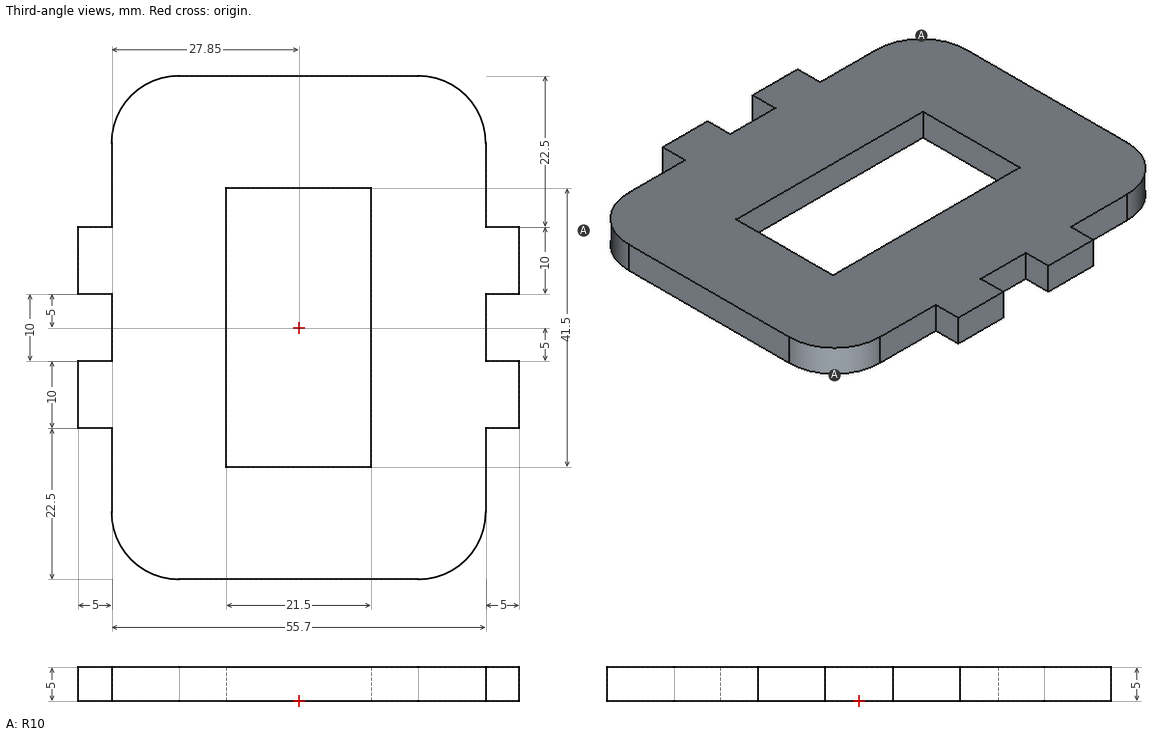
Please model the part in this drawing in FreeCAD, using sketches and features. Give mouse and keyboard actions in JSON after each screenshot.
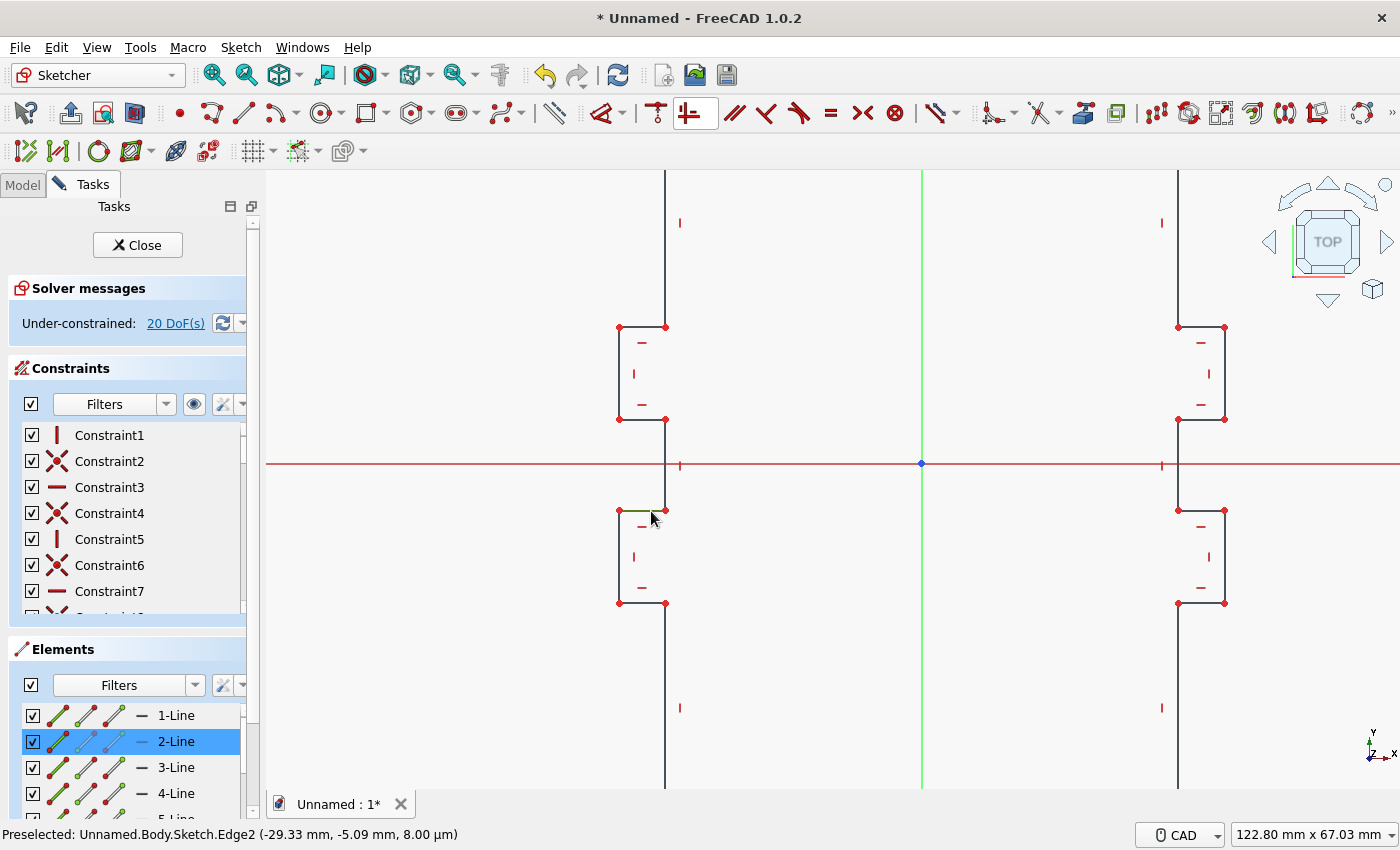
{"action": "key", "text": "l"}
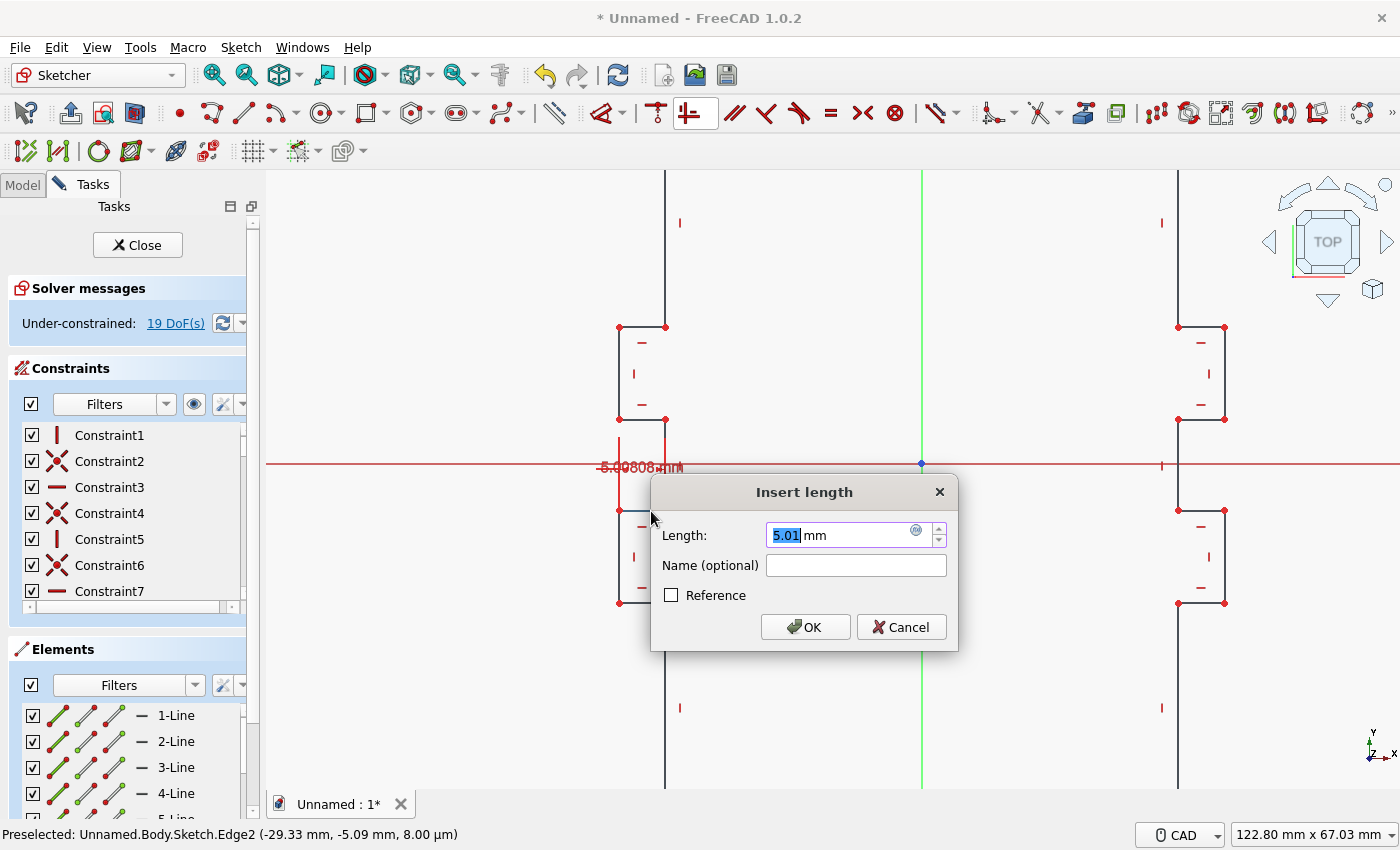
{"action": "type", "text": "5"}
{"action": "key", "text": "Return"}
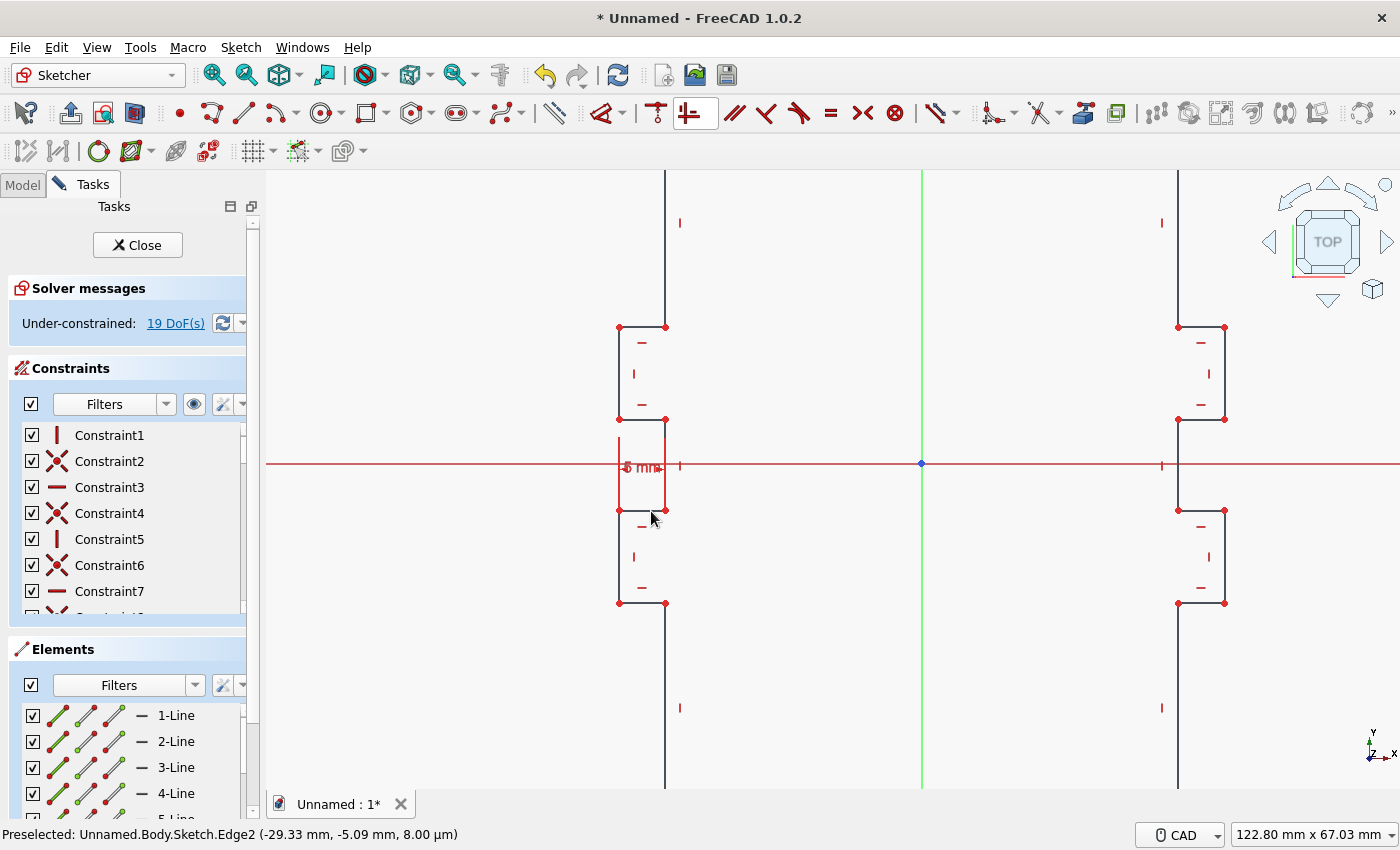
{"action": "left_click", "coordinate": [633, 603]}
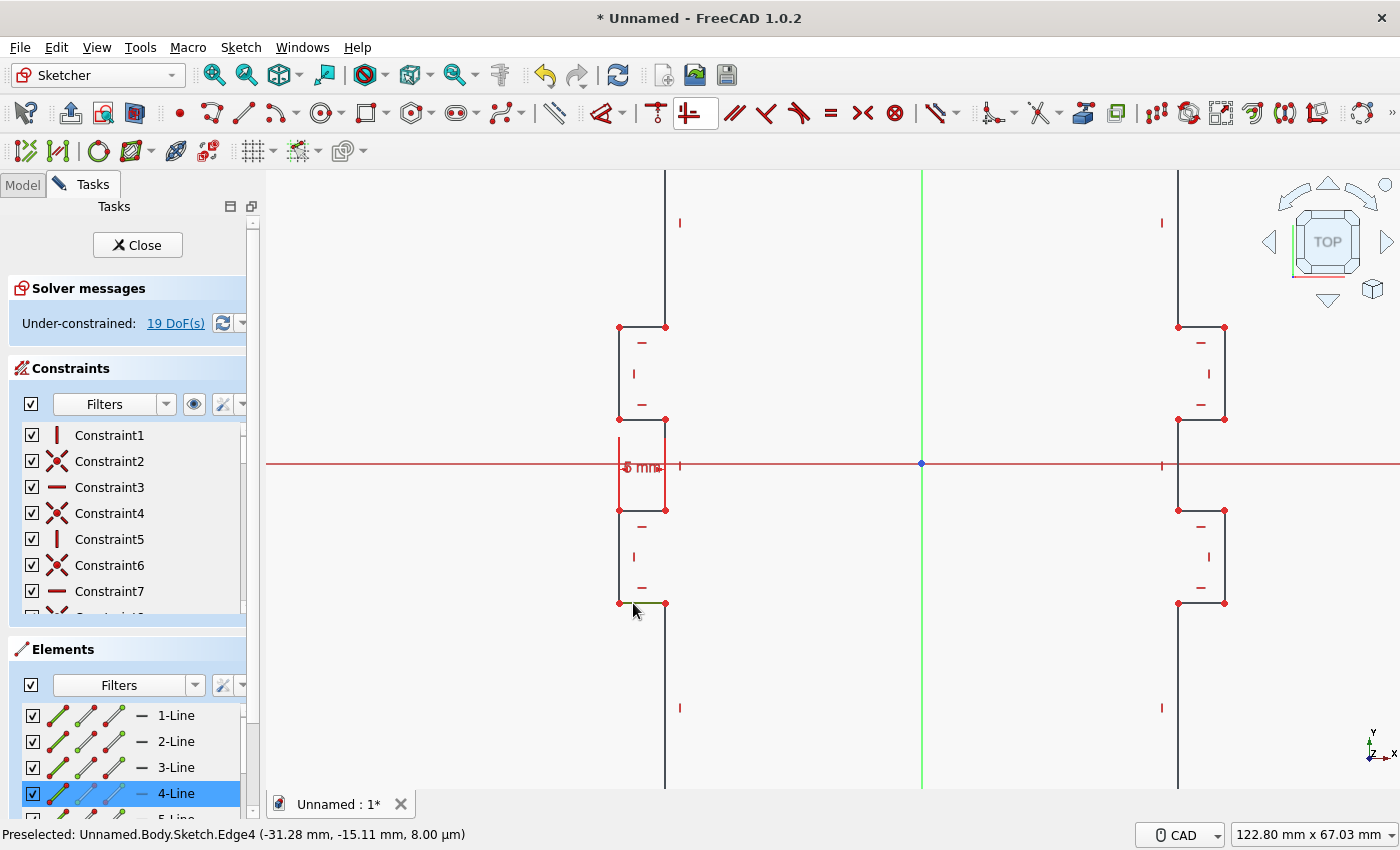
{"action": "left_click", "coordinate": [624, 114]}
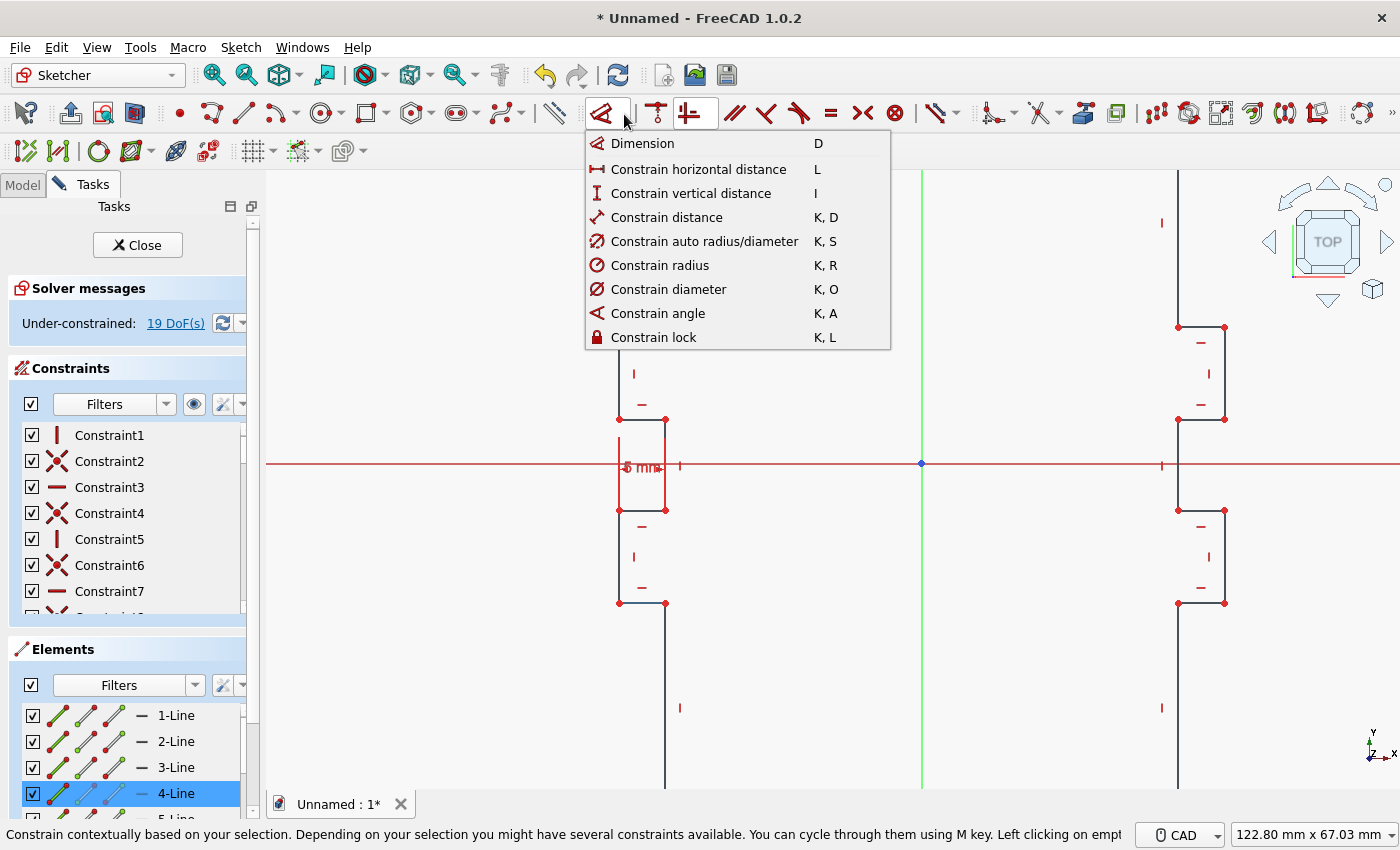
{"action": "left_click", "coordinate": [738, 169]}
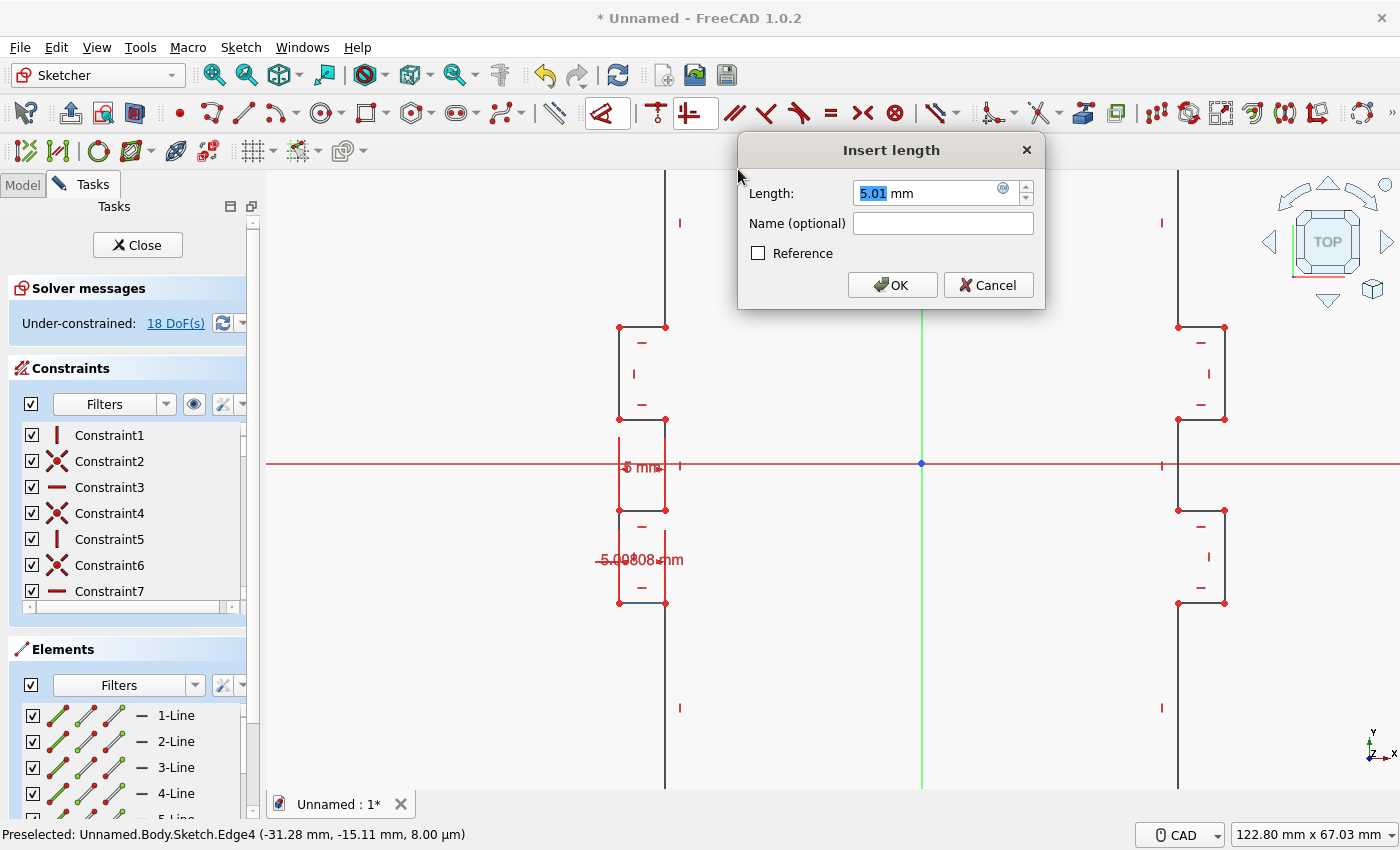
{"action": "type", "text": "5"}
{"action": "key", "text": "Return"}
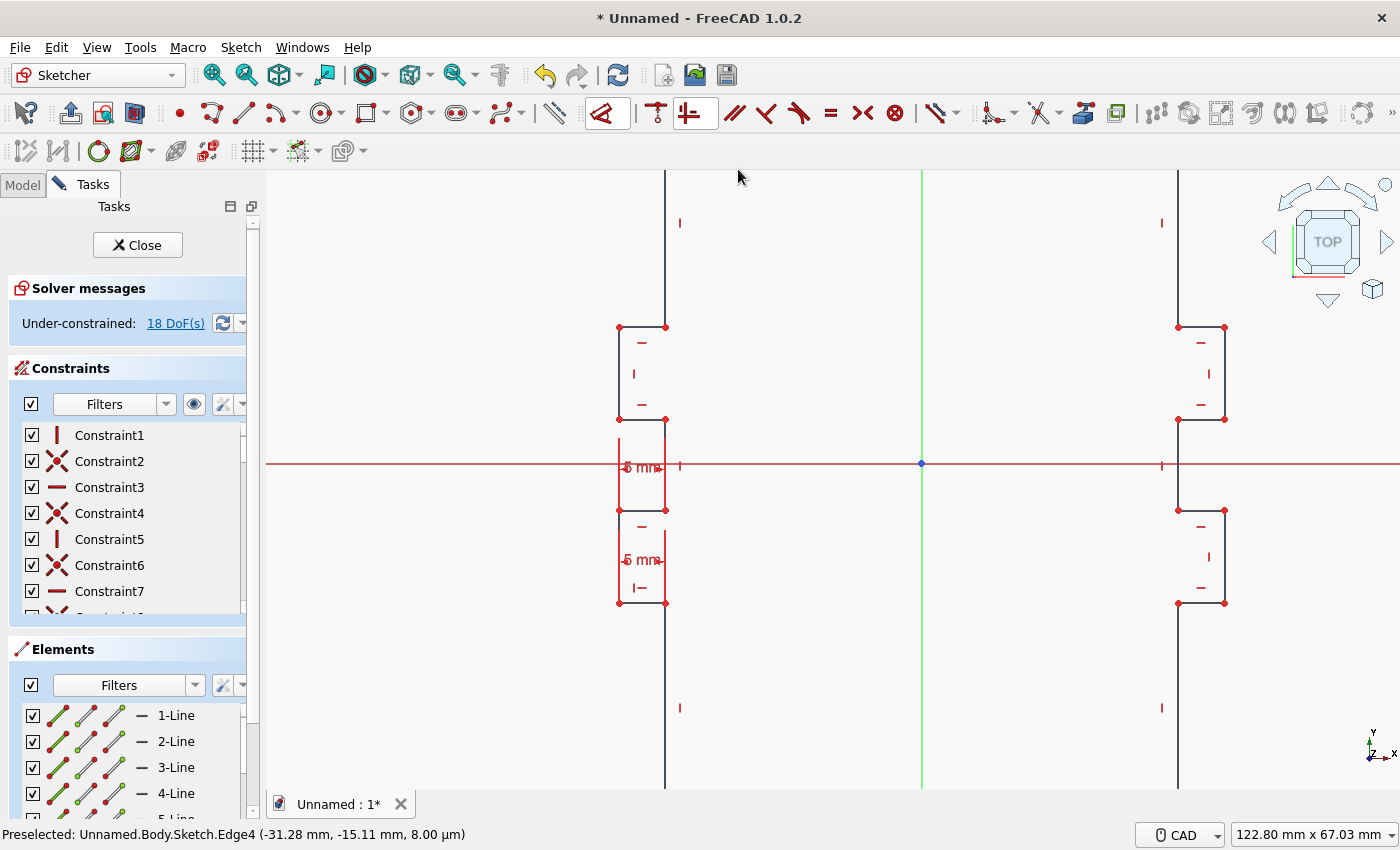
{"action": "left_click", "coordinate": [1192, 603]}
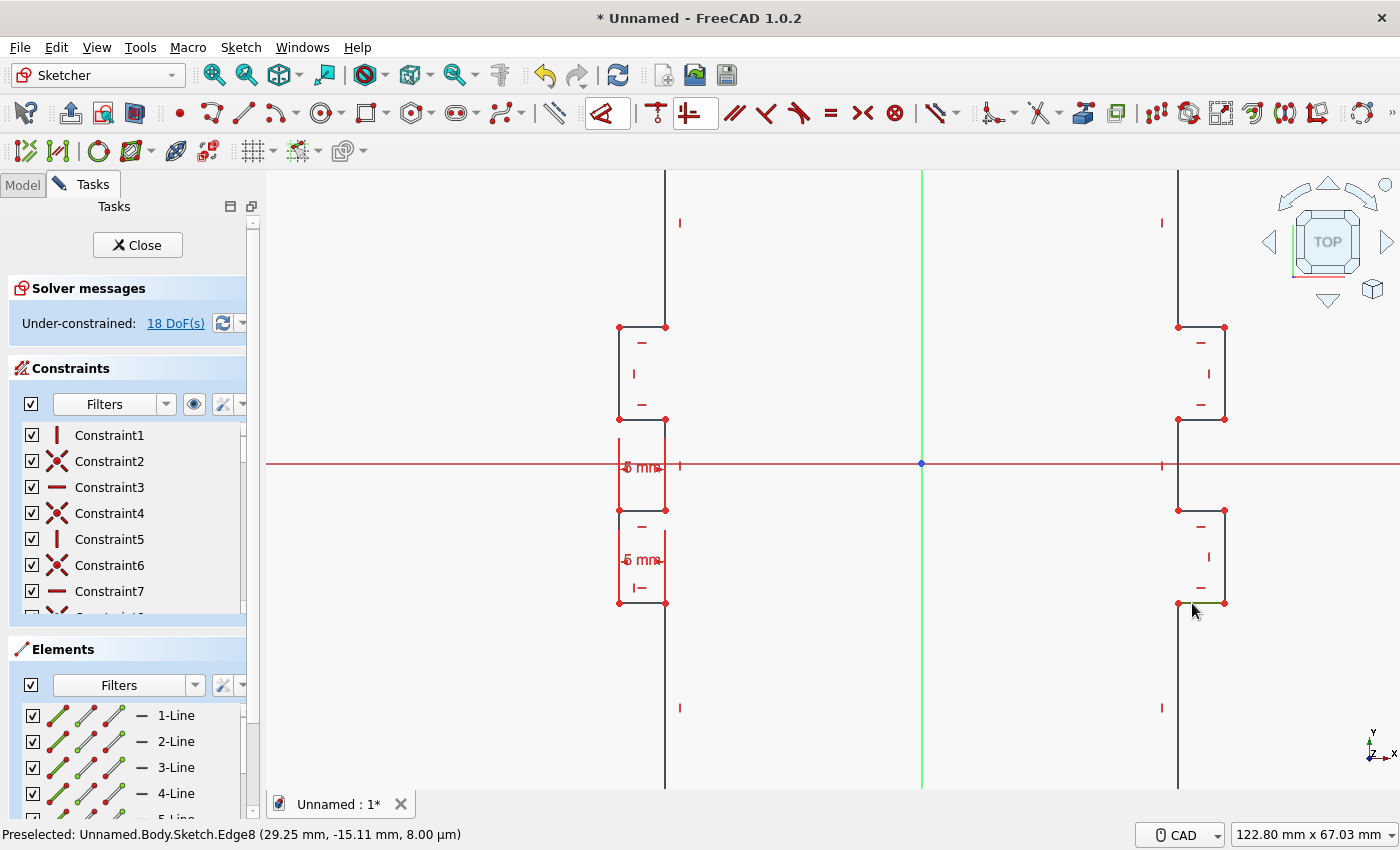
{"action": "key", "text": "l"}